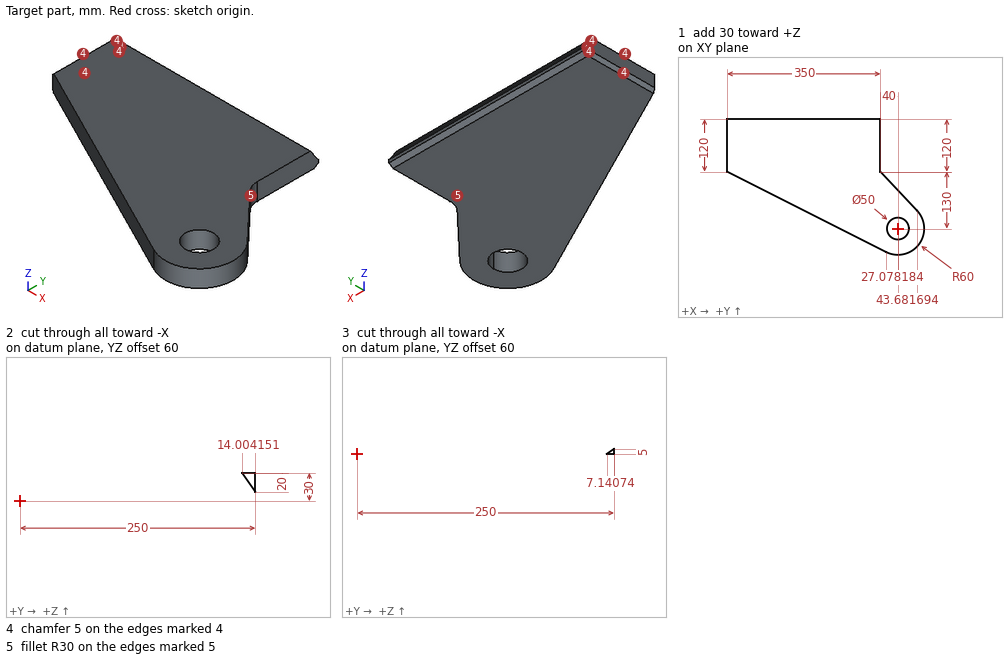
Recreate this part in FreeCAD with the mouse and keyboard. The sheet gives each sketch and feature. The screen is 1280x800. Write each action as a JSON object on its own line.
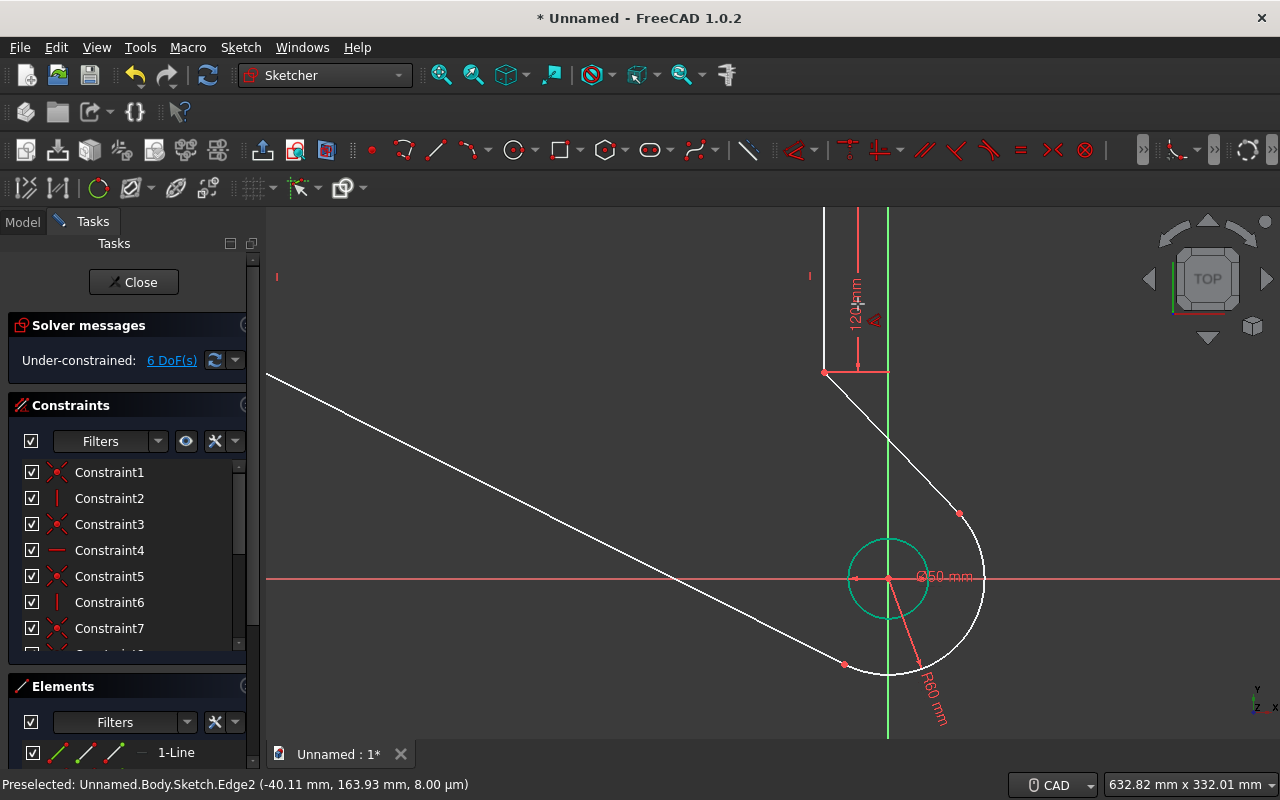
{"action": "scroll", "coordinate": [888, 578], "scroll_direction": "down", "scroll_amount": 2}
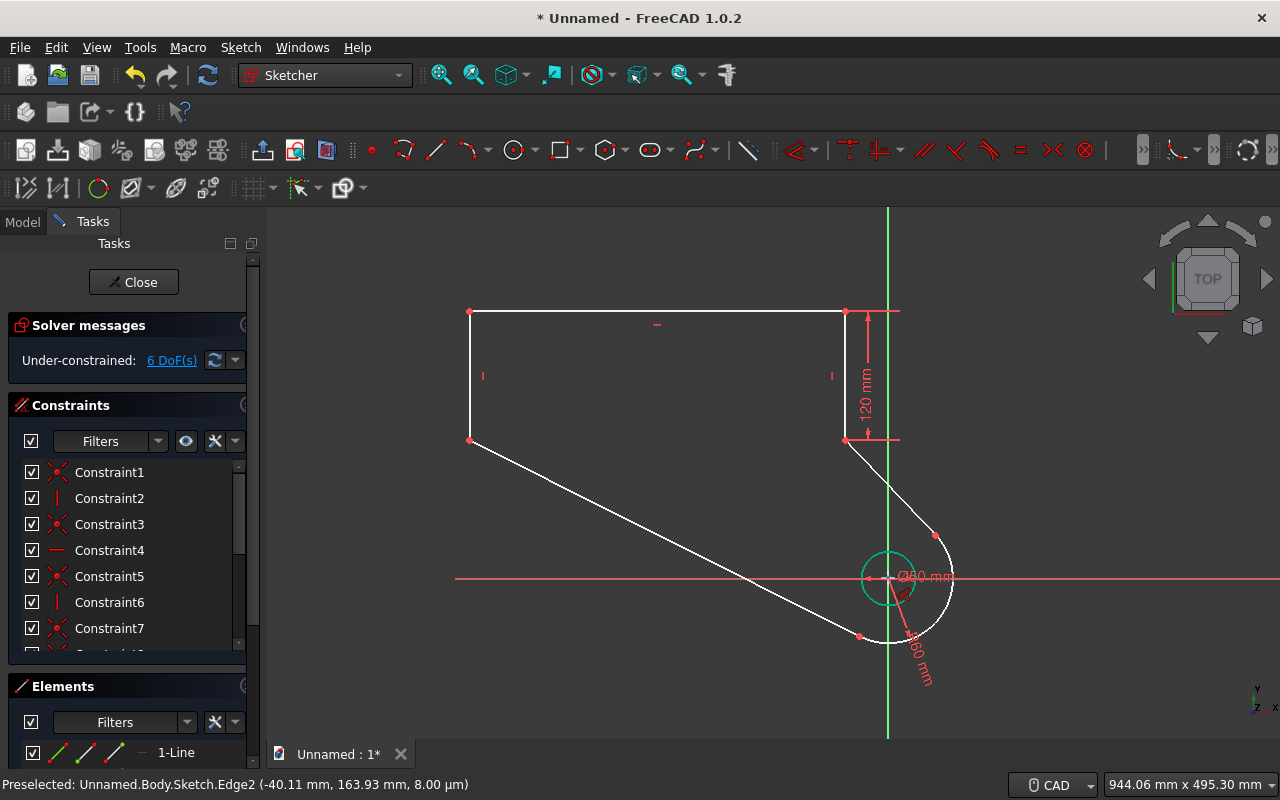
{"action": "left_click", "coordinate": [733, 311]}
{"action": "left_click", "coordinate": [658, 277]}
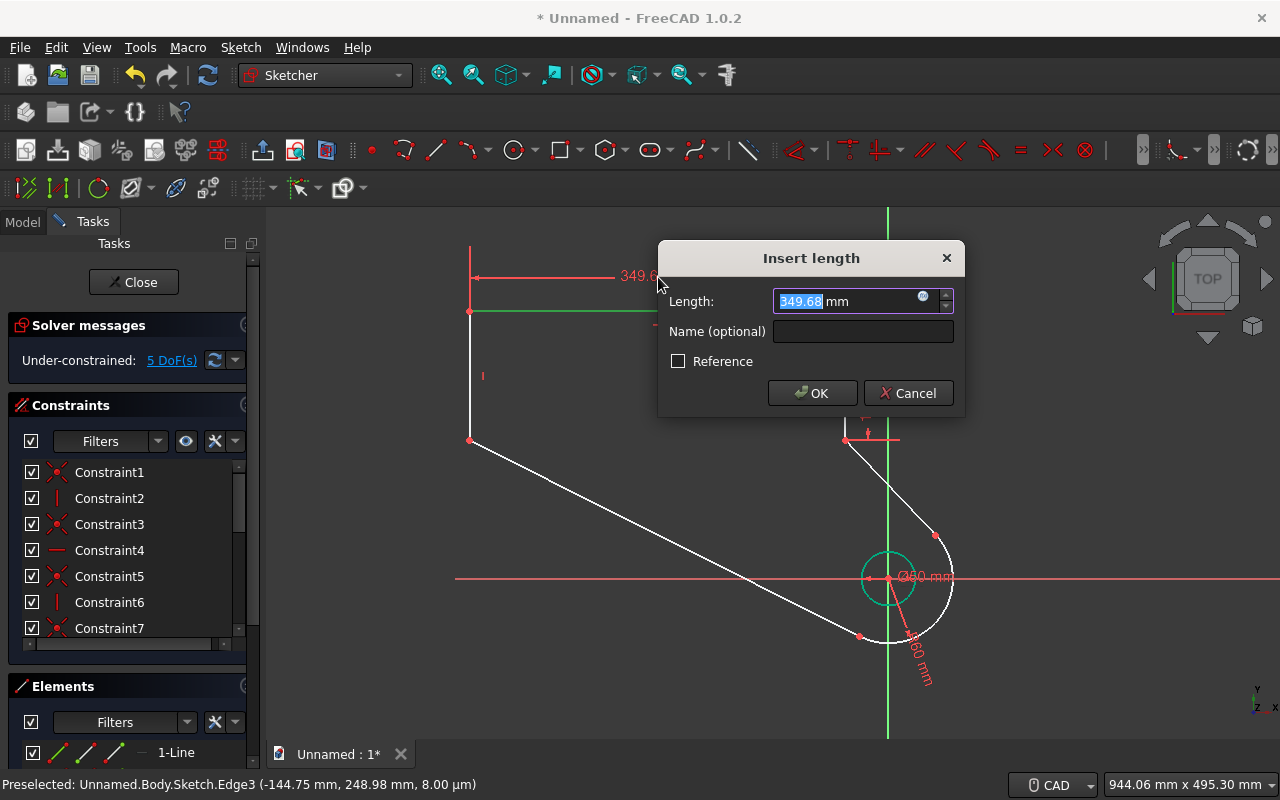
{"action": "type", "text": "350"}
{"action": "key", "text": "Return"}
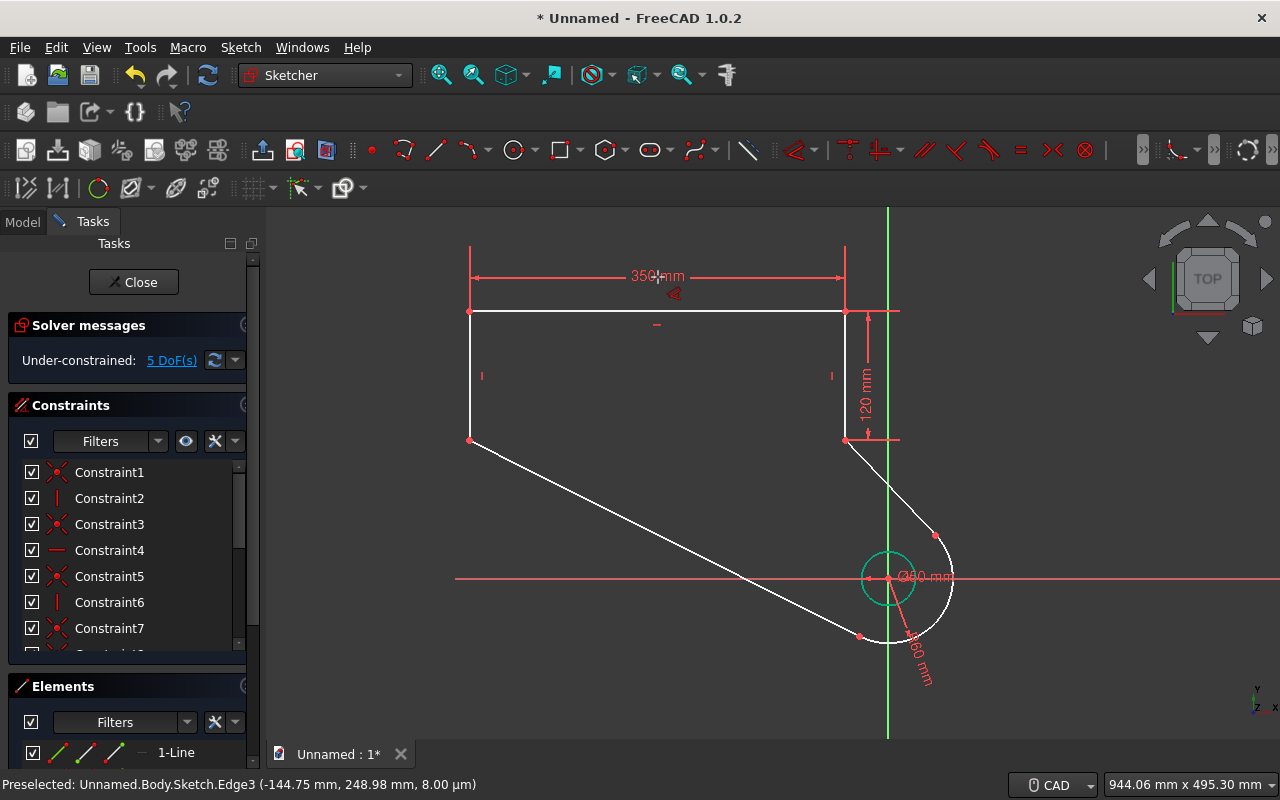
{"action": "left_click", "coordinate": [470, 350]}
{"action": "left_click", "coordinate": [436, 376]}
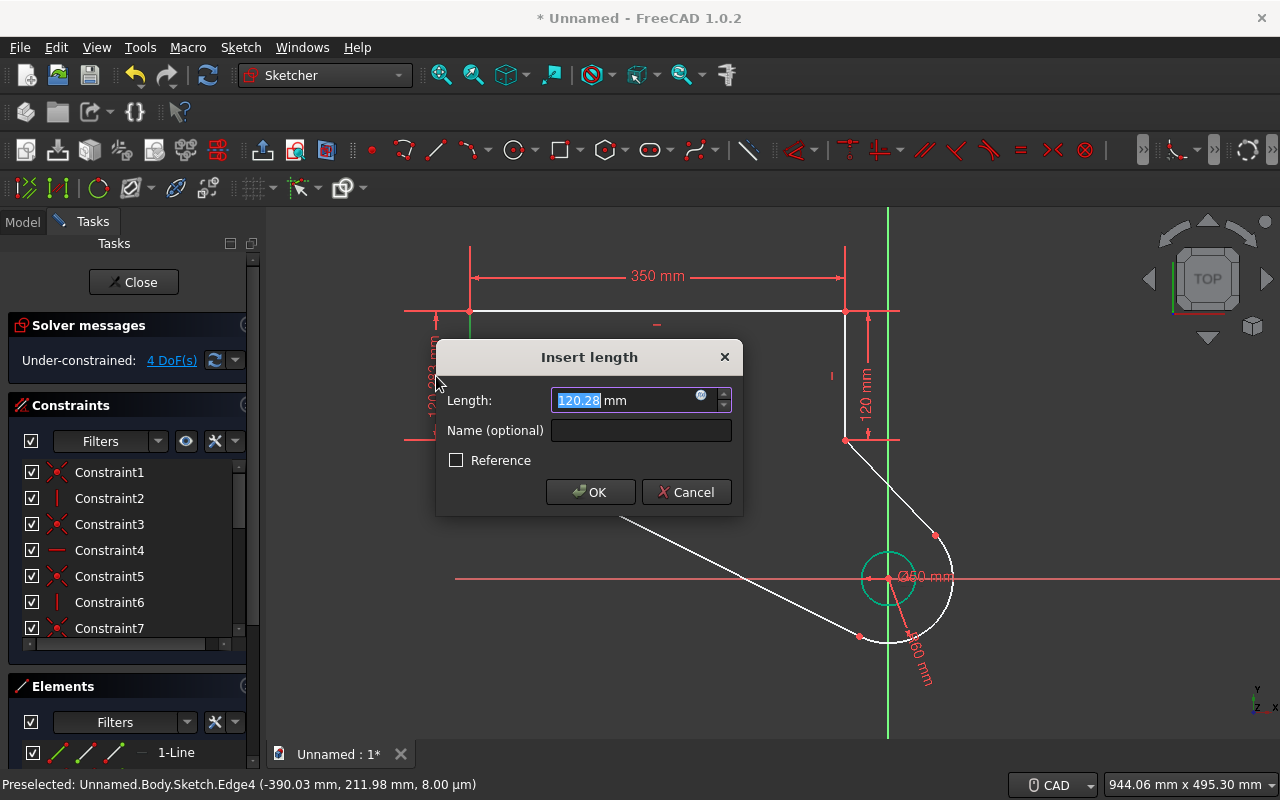
{"action": "type", "text": "120"}
{"action": "key", "text": "Return"}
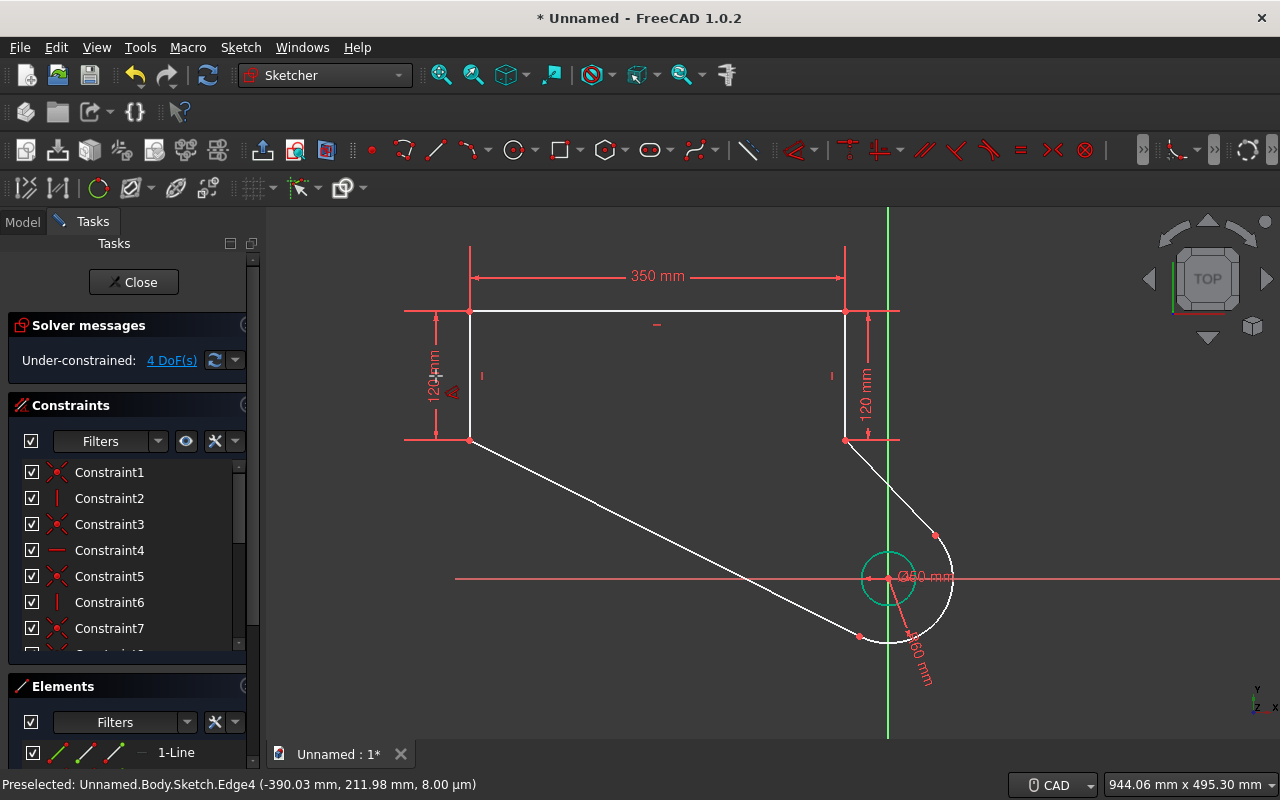
{"action": "left_click", "coordinate": [845, 440]}
{"action": "left_click", "coordinate": [867, 613]}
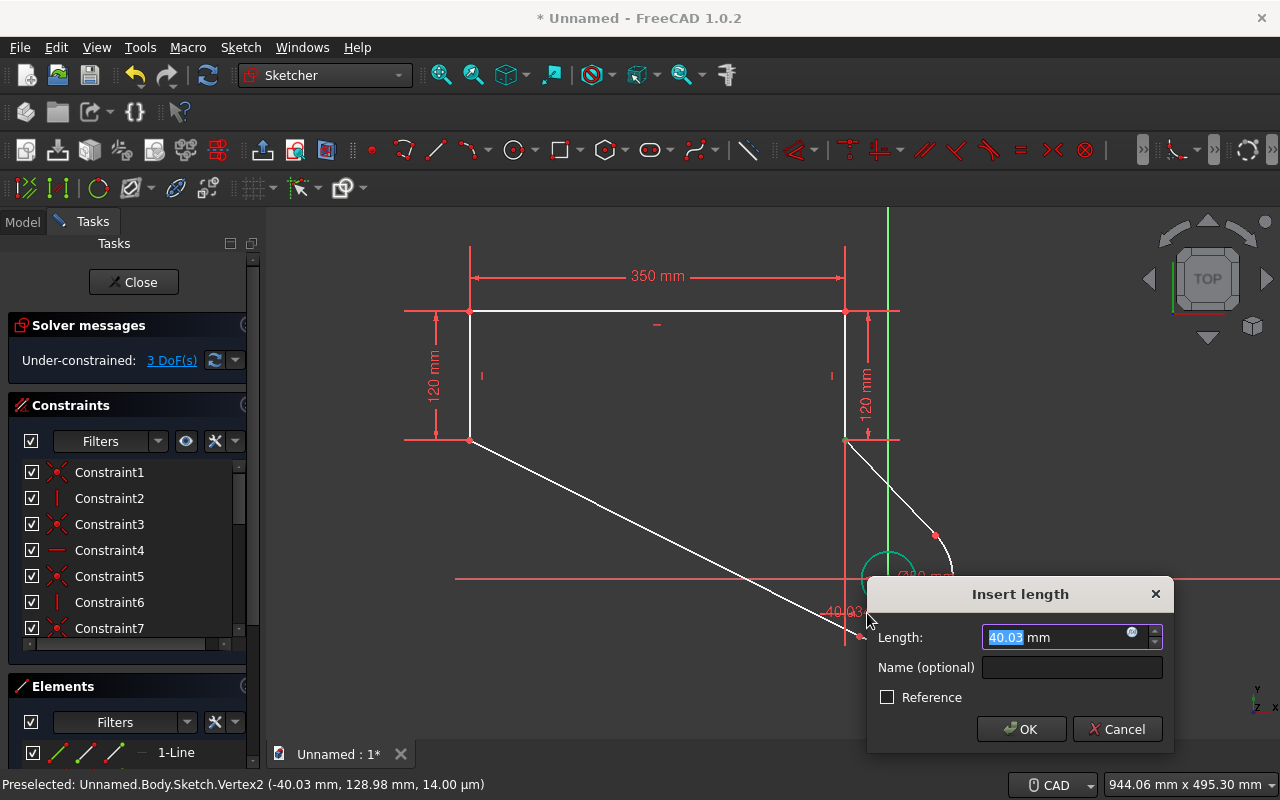
{"action": "type", "text": "40"}
{"action": "key", "text": "Return"}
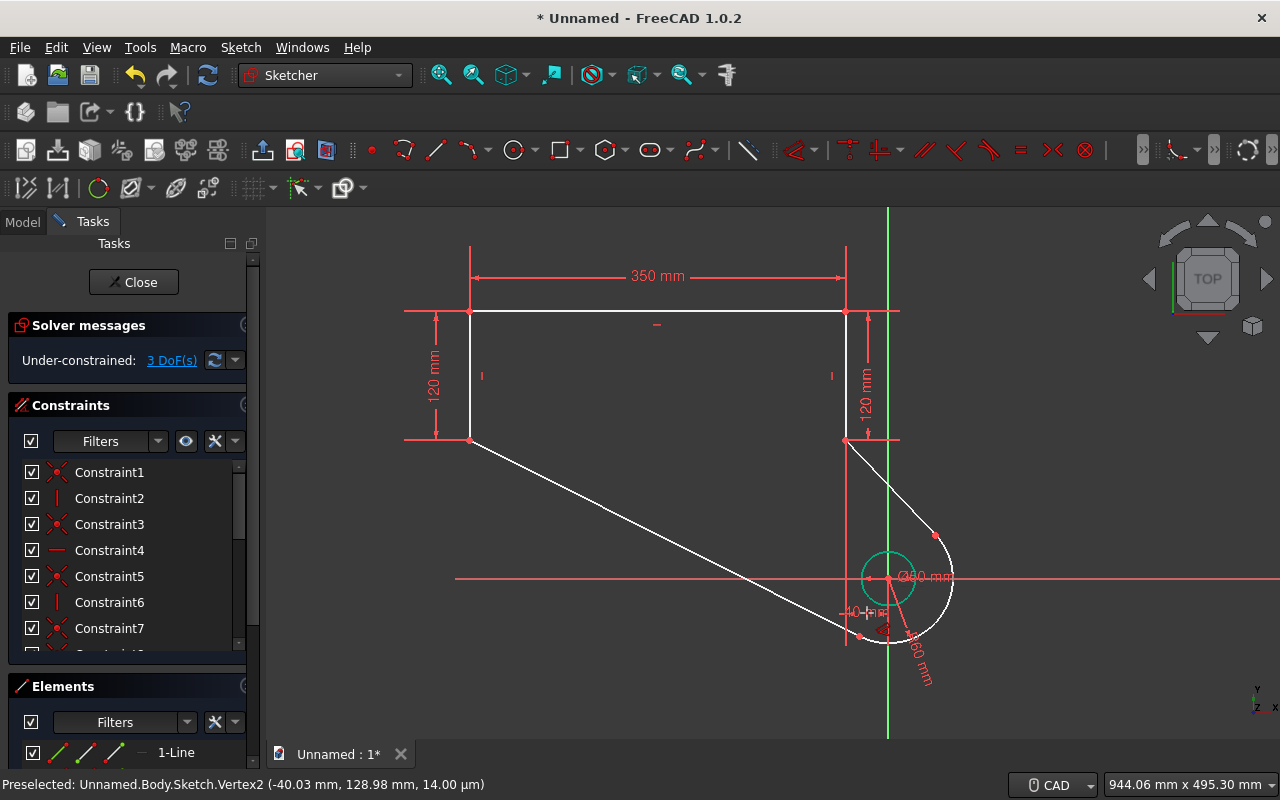
{"action": "left_click", "coordinate": [846, 440]}
{"action": "left_click", "coordinate": [922, 478]}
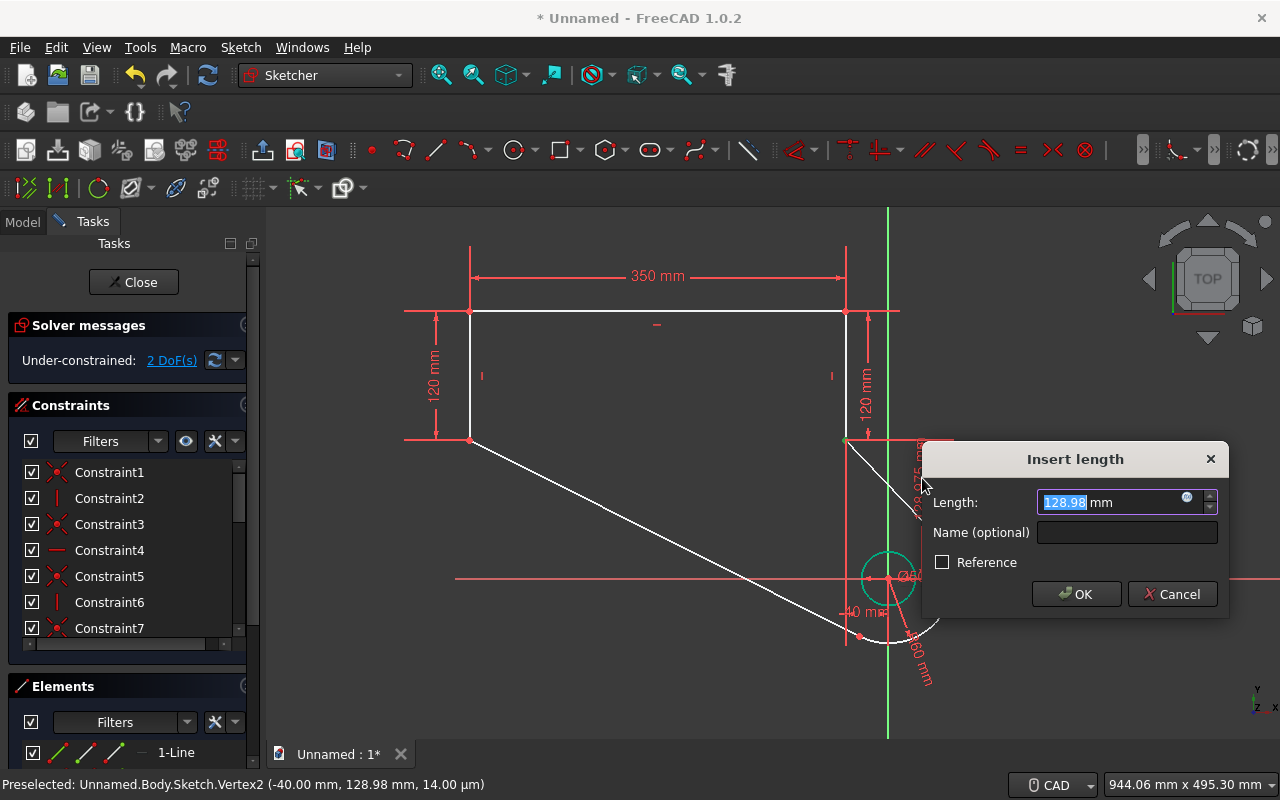
{"action": "type", "text": "130"}
{"action": "key", "text": "Return"}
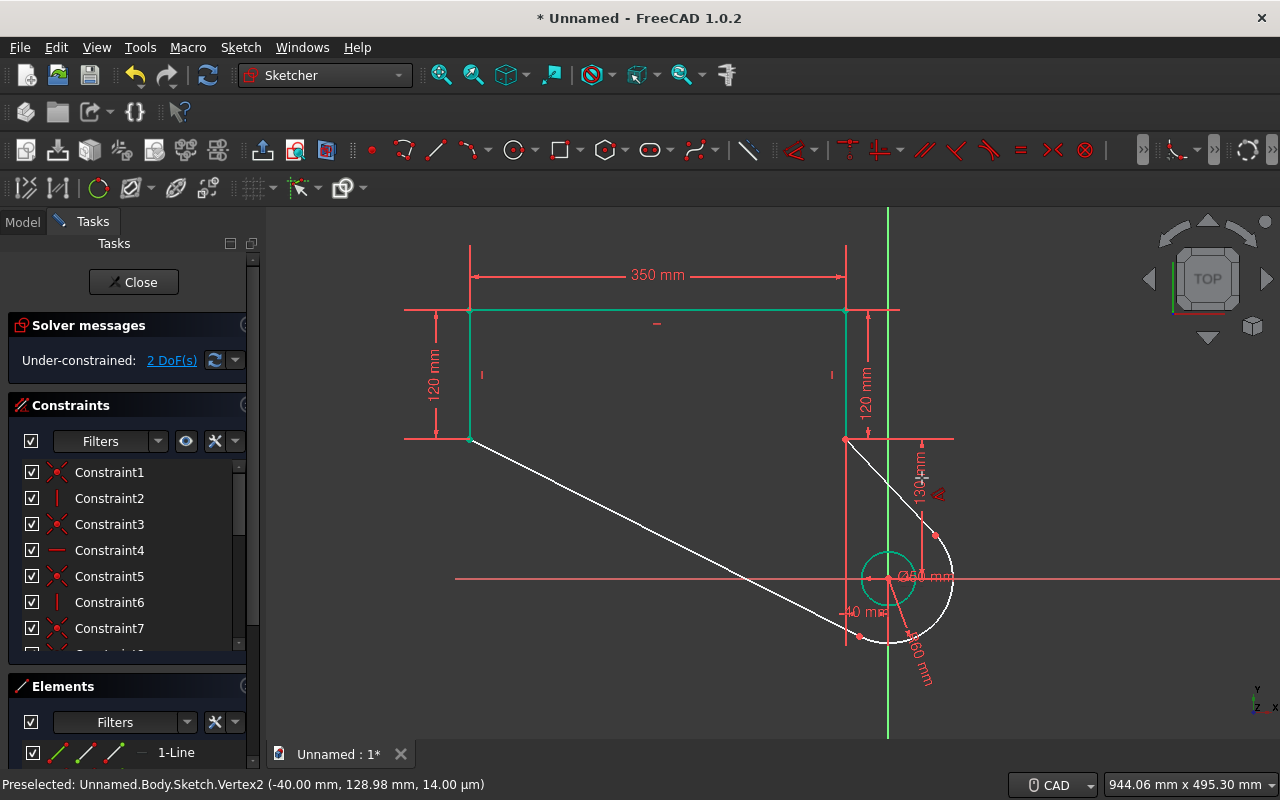
{"action": "left_click", "coordinate": [936, 535]}
{"action": "left_click", "coordinate": [923, 501]}